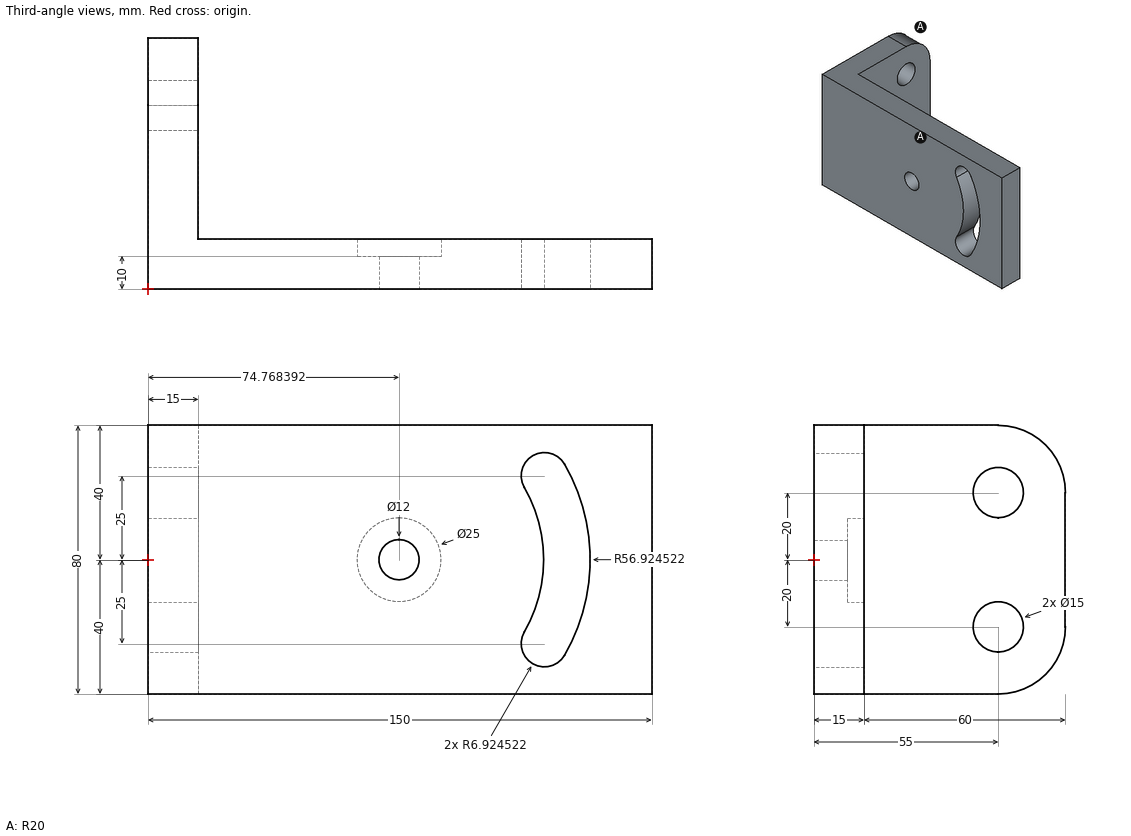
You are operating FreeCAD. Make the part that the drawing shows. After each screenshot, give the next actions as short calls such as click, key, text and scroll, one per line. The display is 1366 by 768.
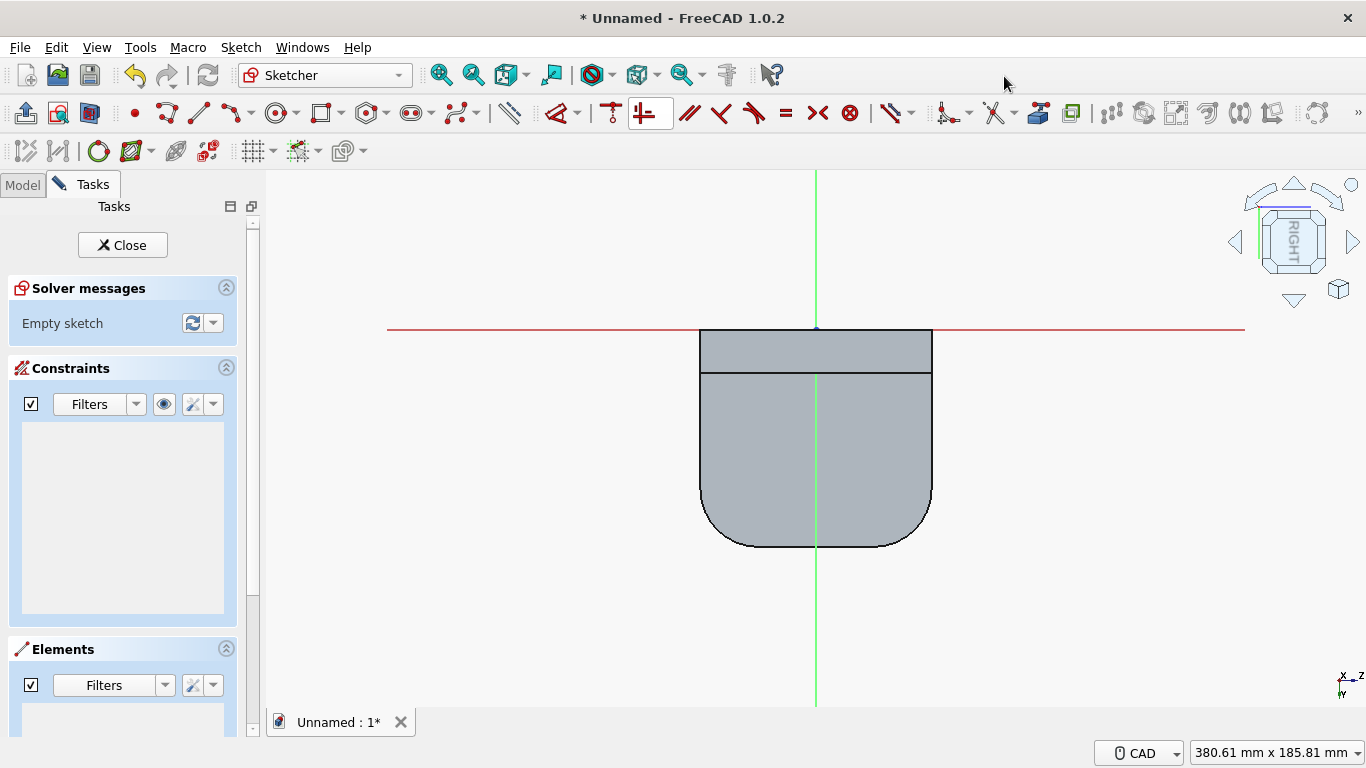
scroll(899, 398, up, 3)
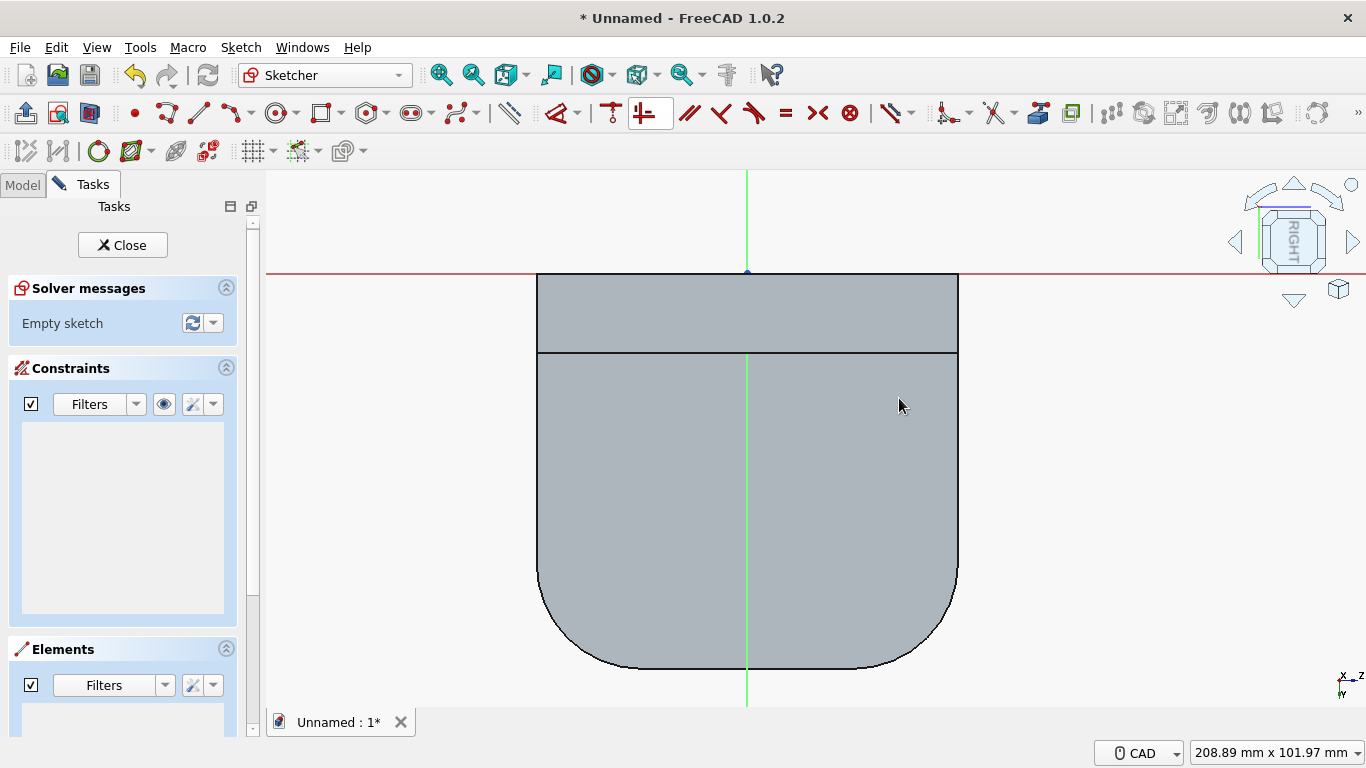
key(g)
key(c)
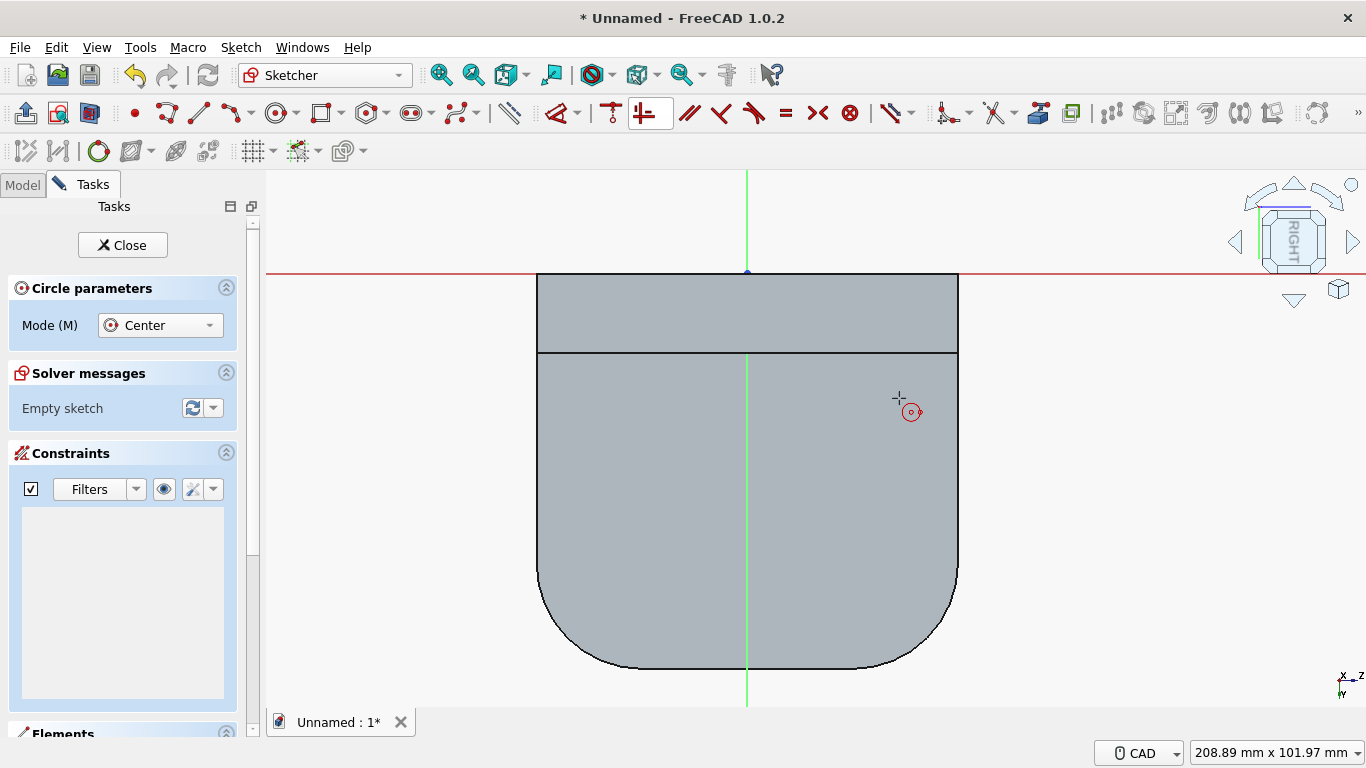
click(642, 564)
click(670, 536)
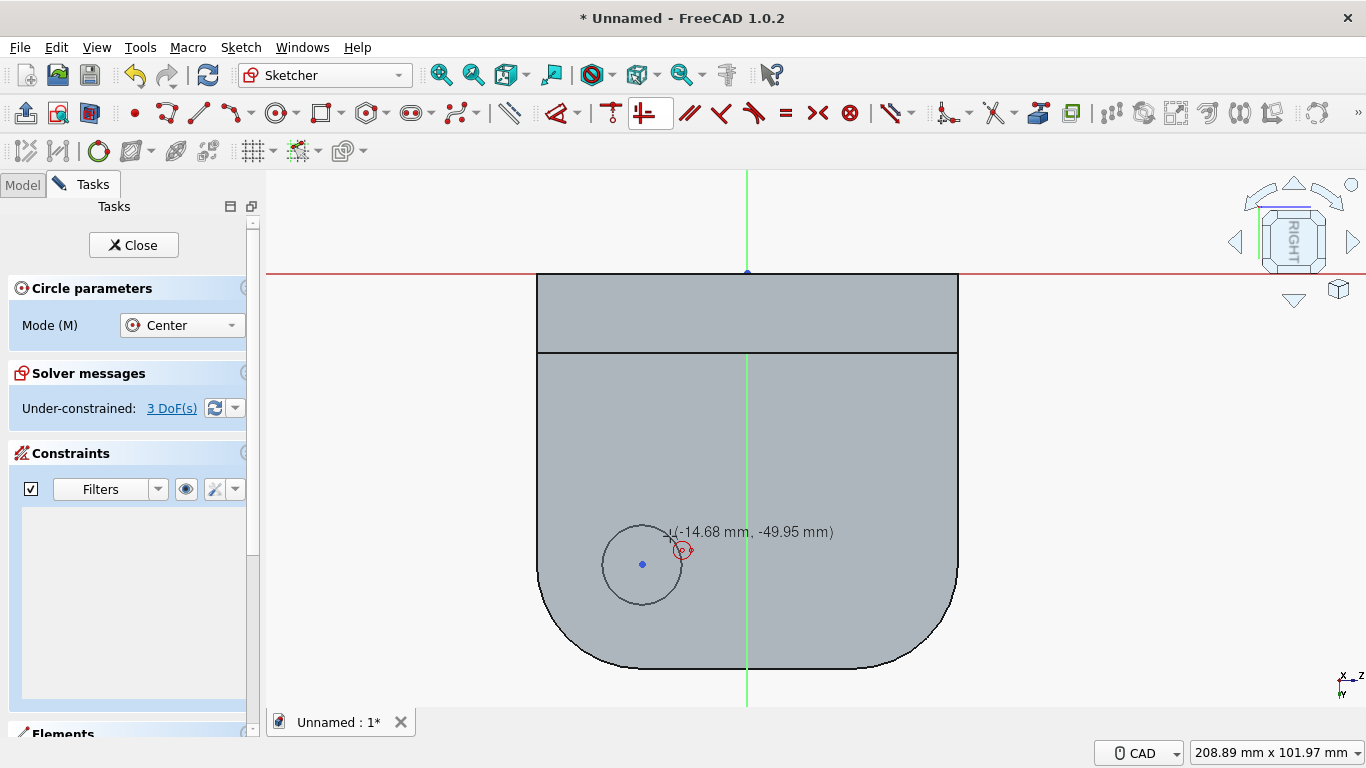
click(853, 564)
click(881, 536)
key(Escape)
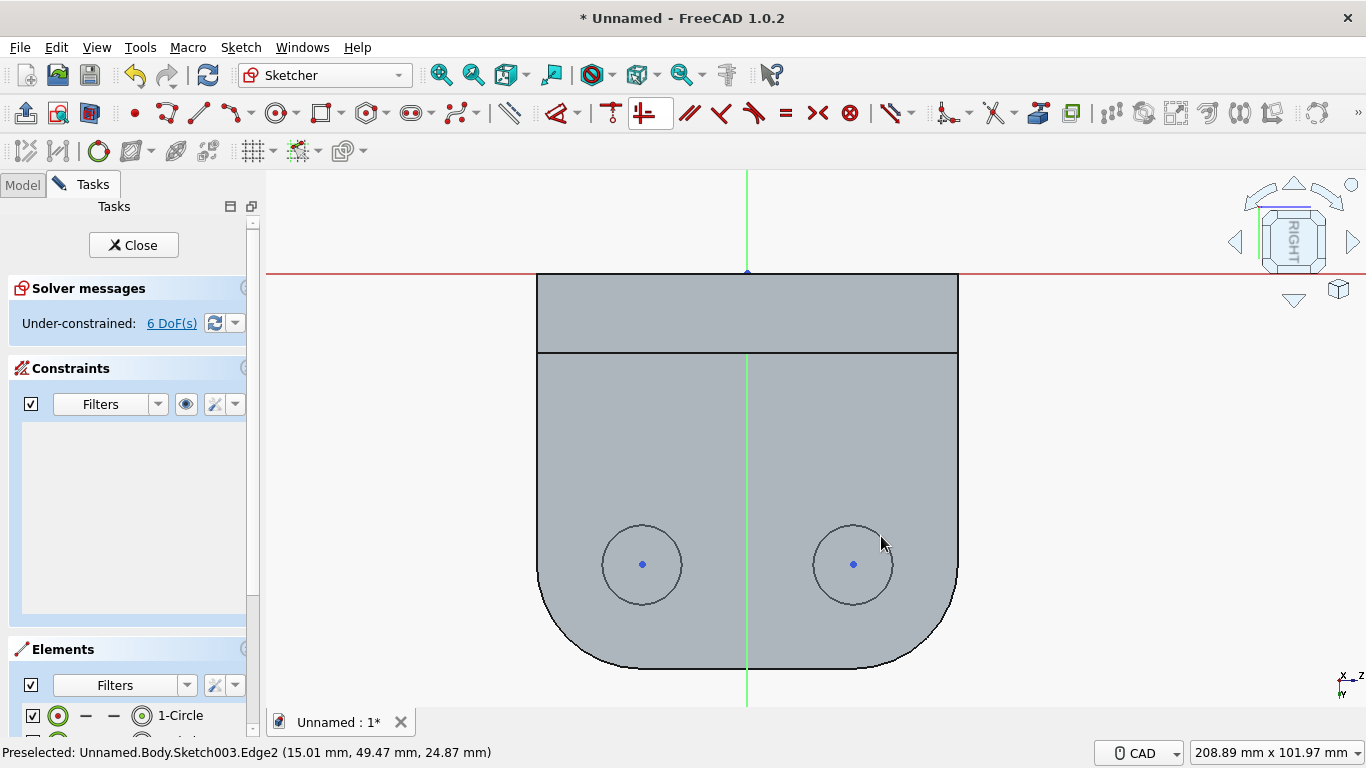
click(670, 537)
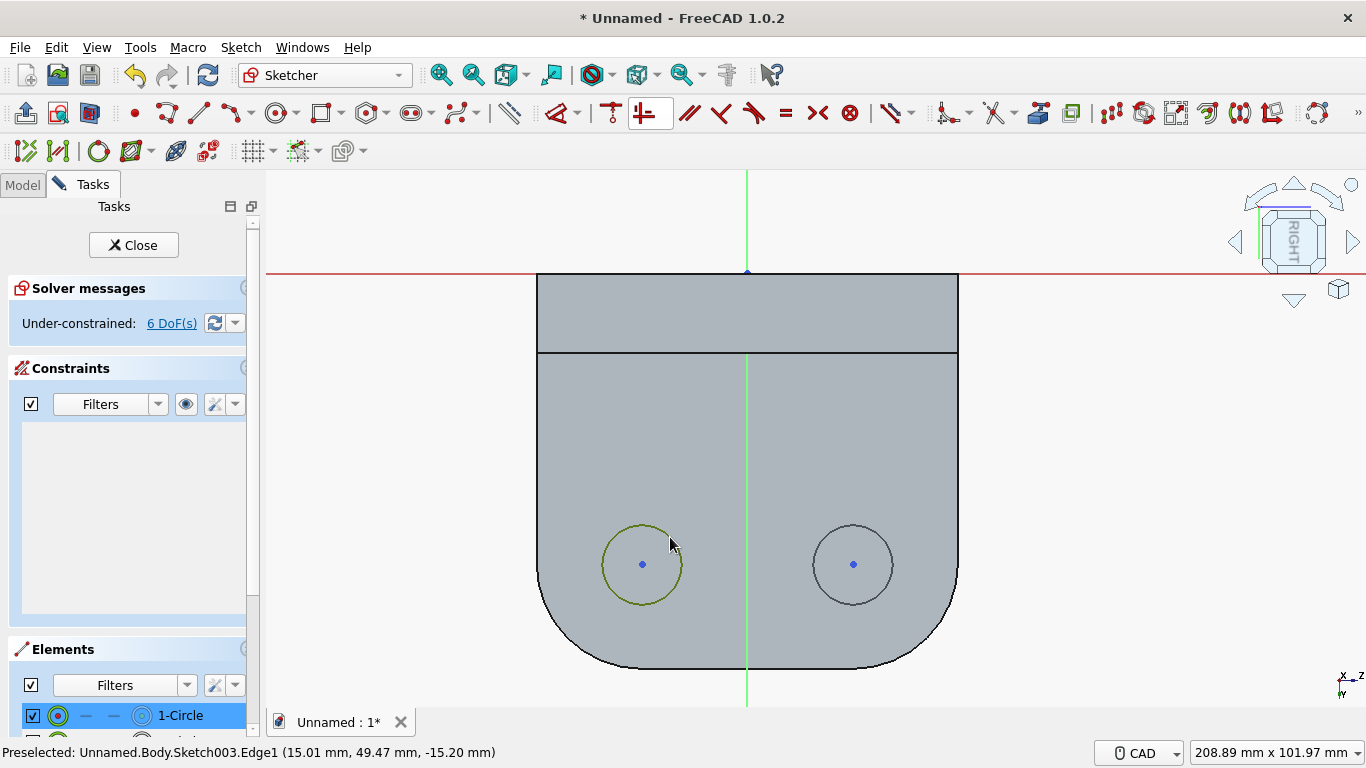
click(881, 537)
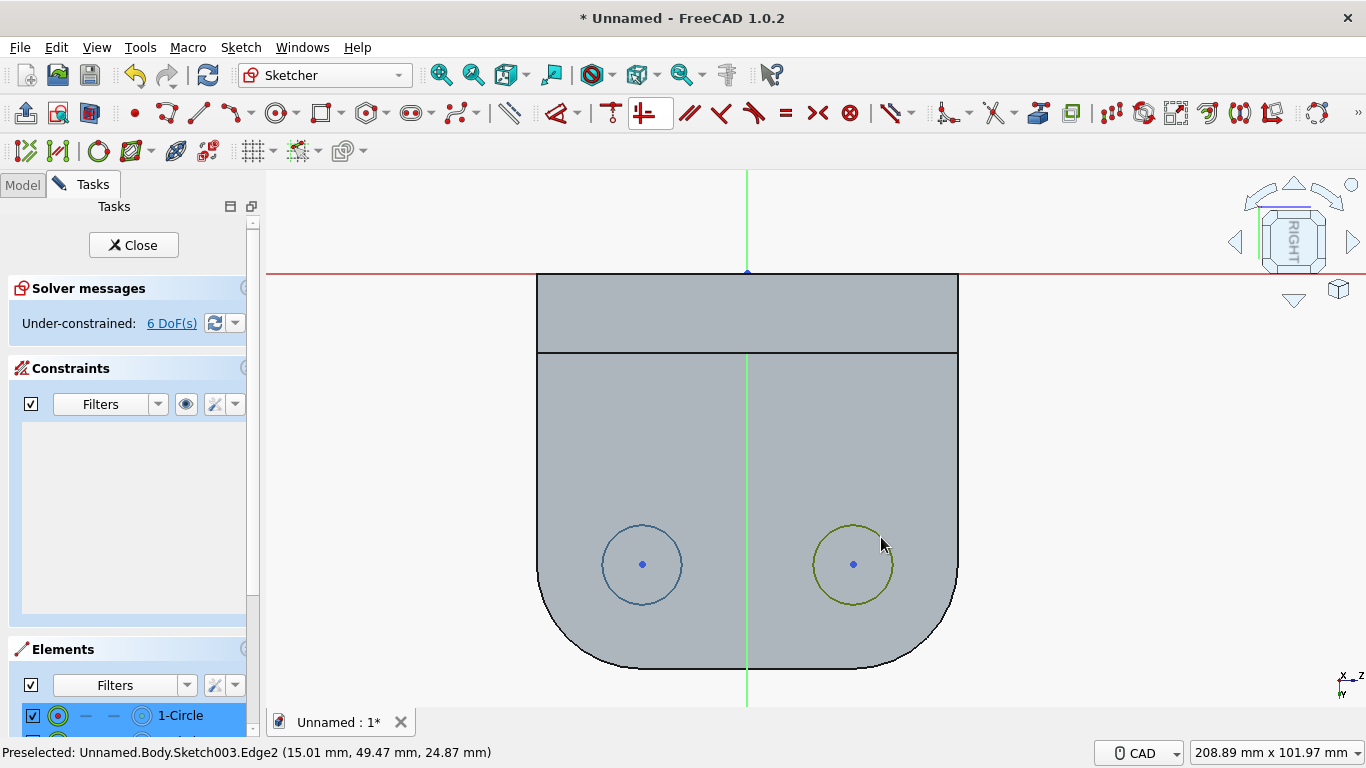
click(786, 114)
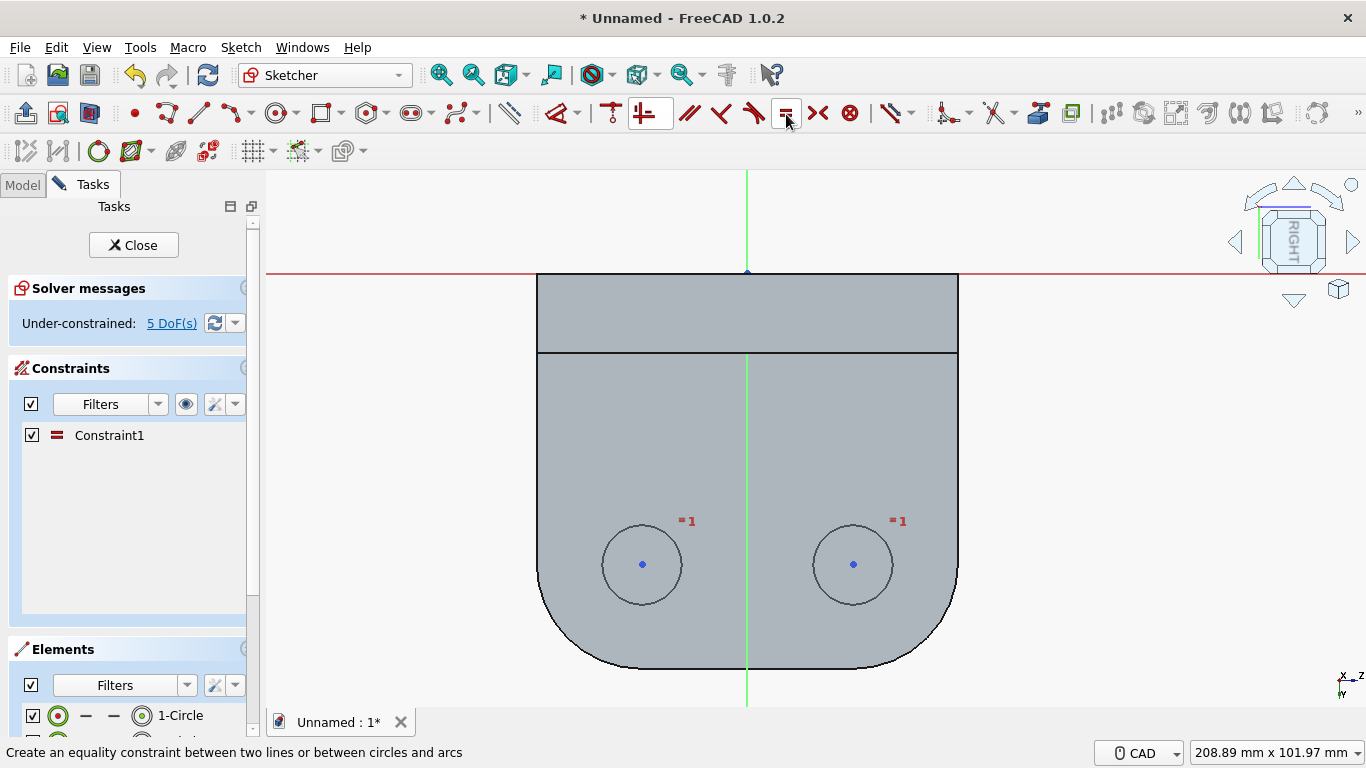
click(642, 565)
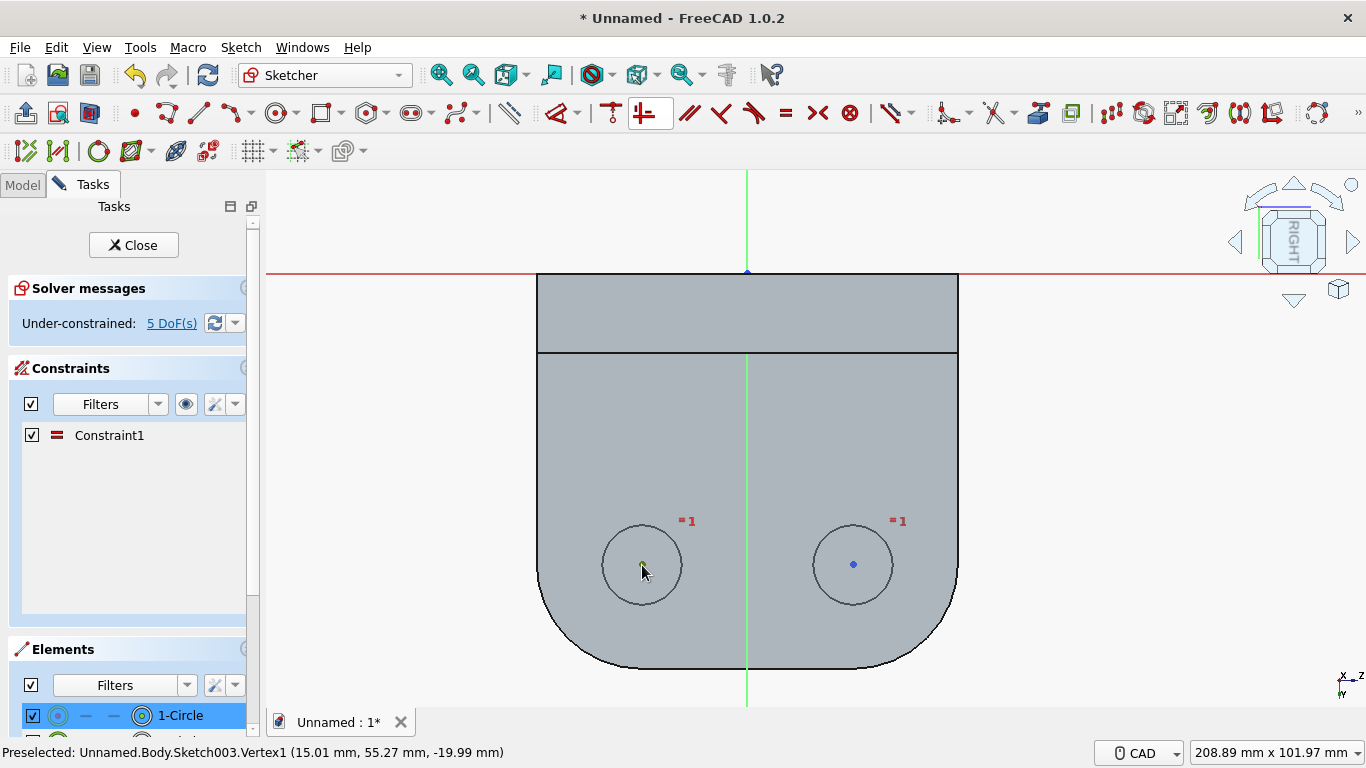
click(853, 565)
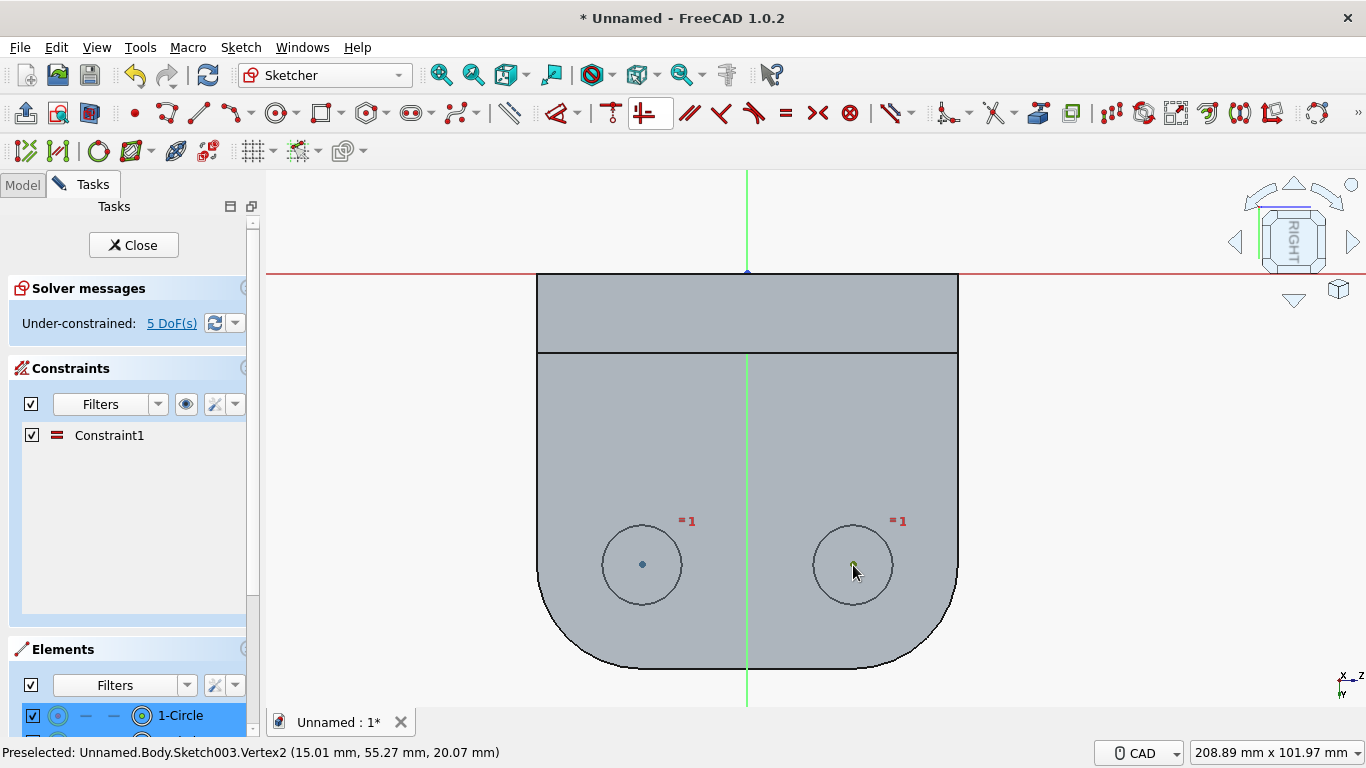
key(h)